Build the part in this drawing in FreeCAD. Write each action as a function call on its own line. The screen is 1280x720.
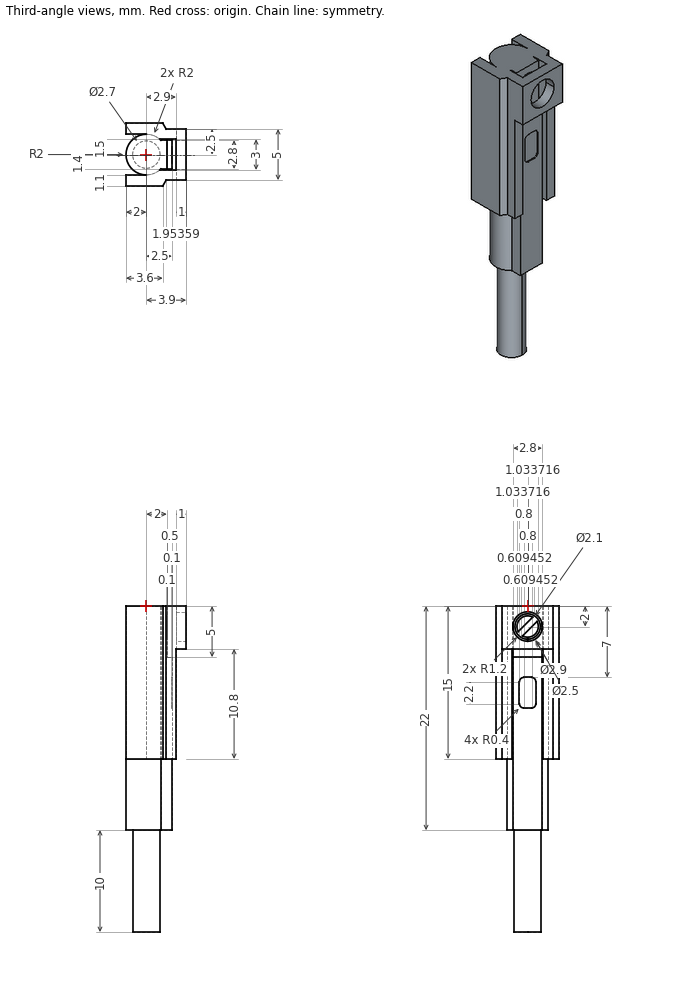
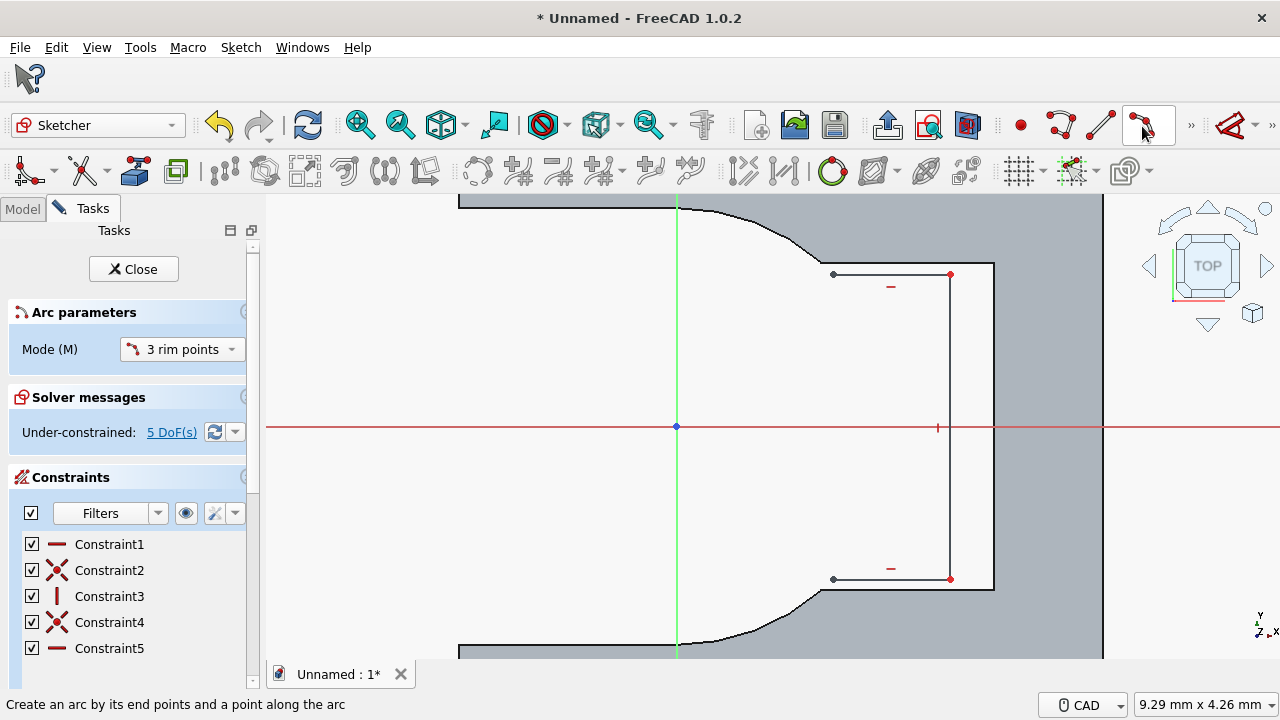
click(833, 275)
click(833, 580)
click(483, 327)
key(Escape)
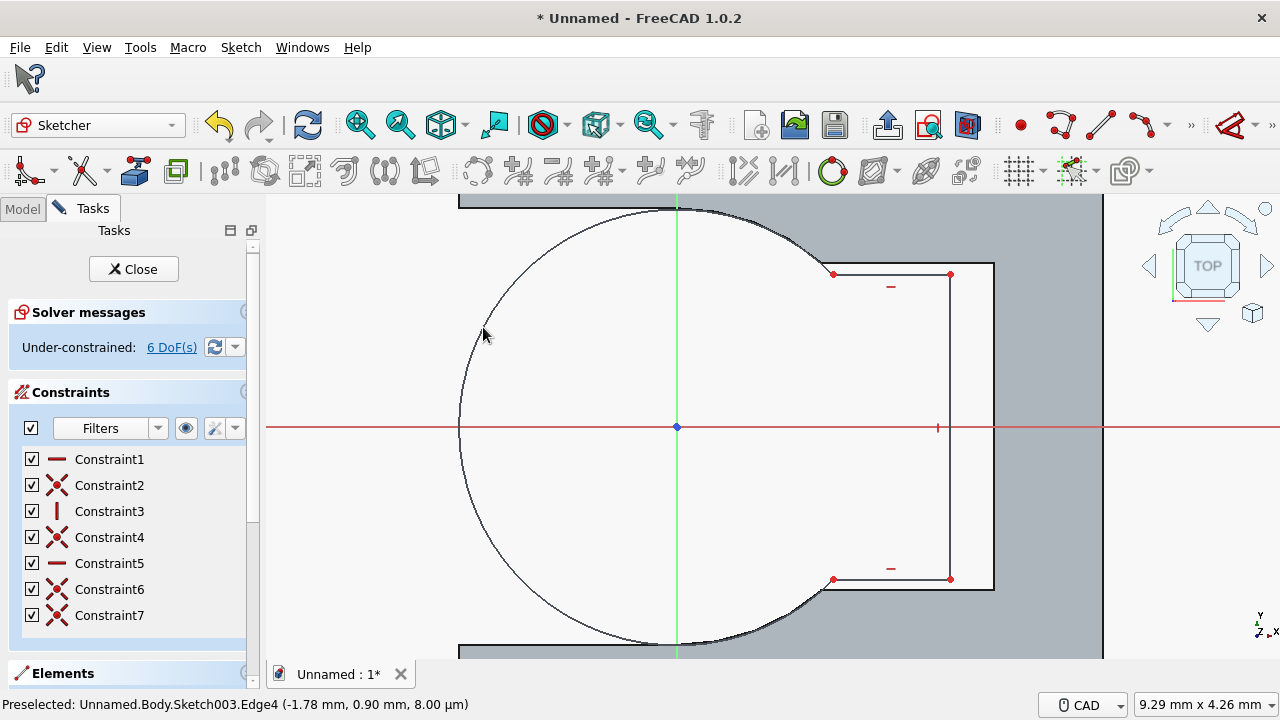
drag(667, 416, 687, 438)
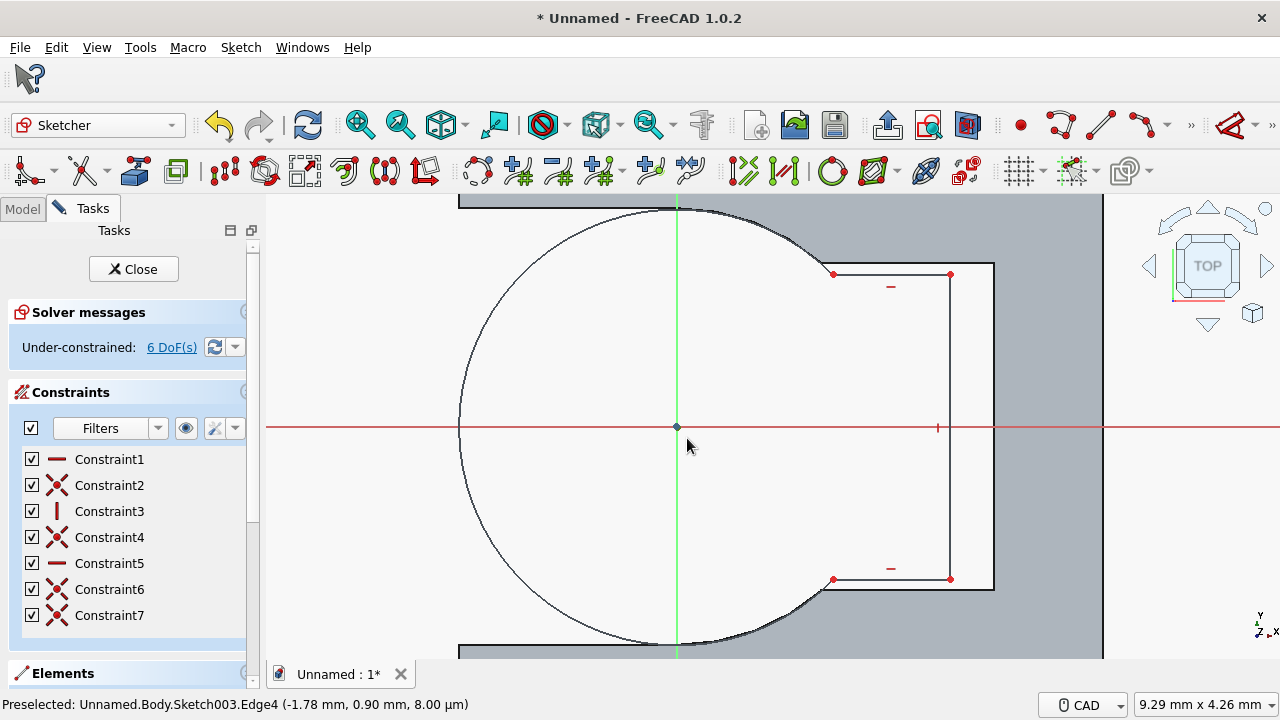
key(c)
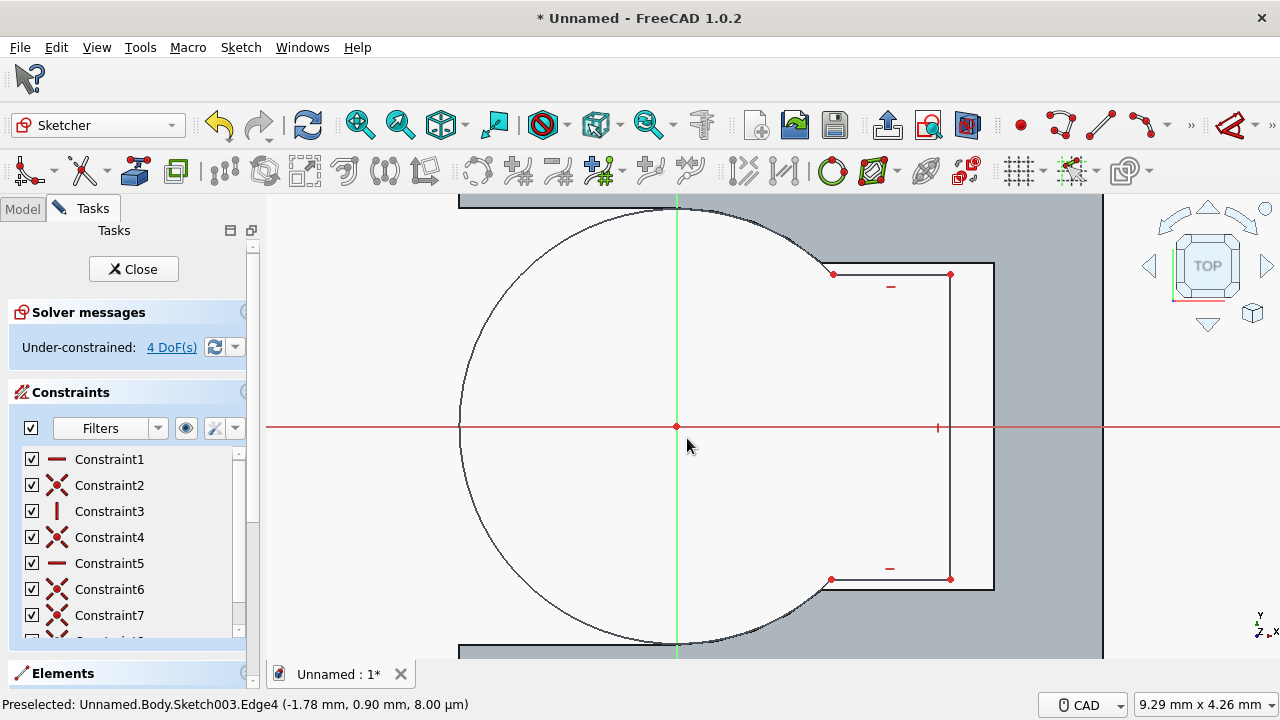
click(1230, 126)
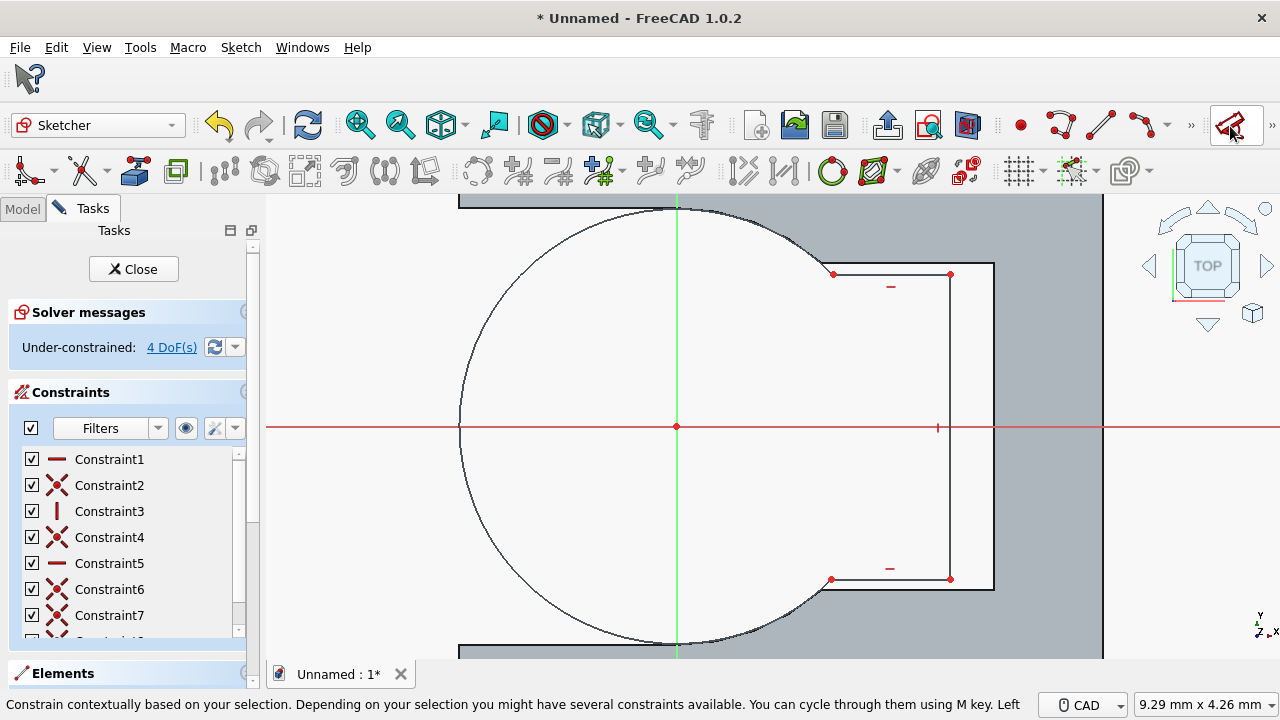
click(551, 249)
click(532, 223)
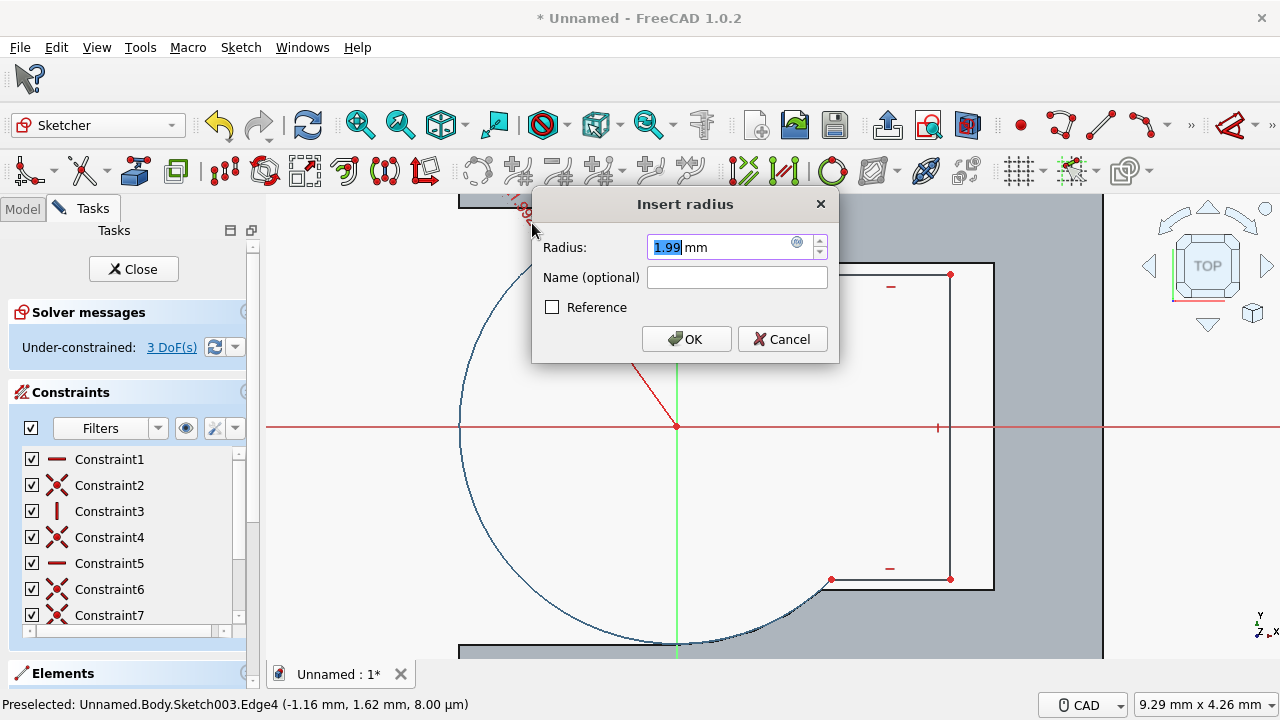
text(2)
key(Return)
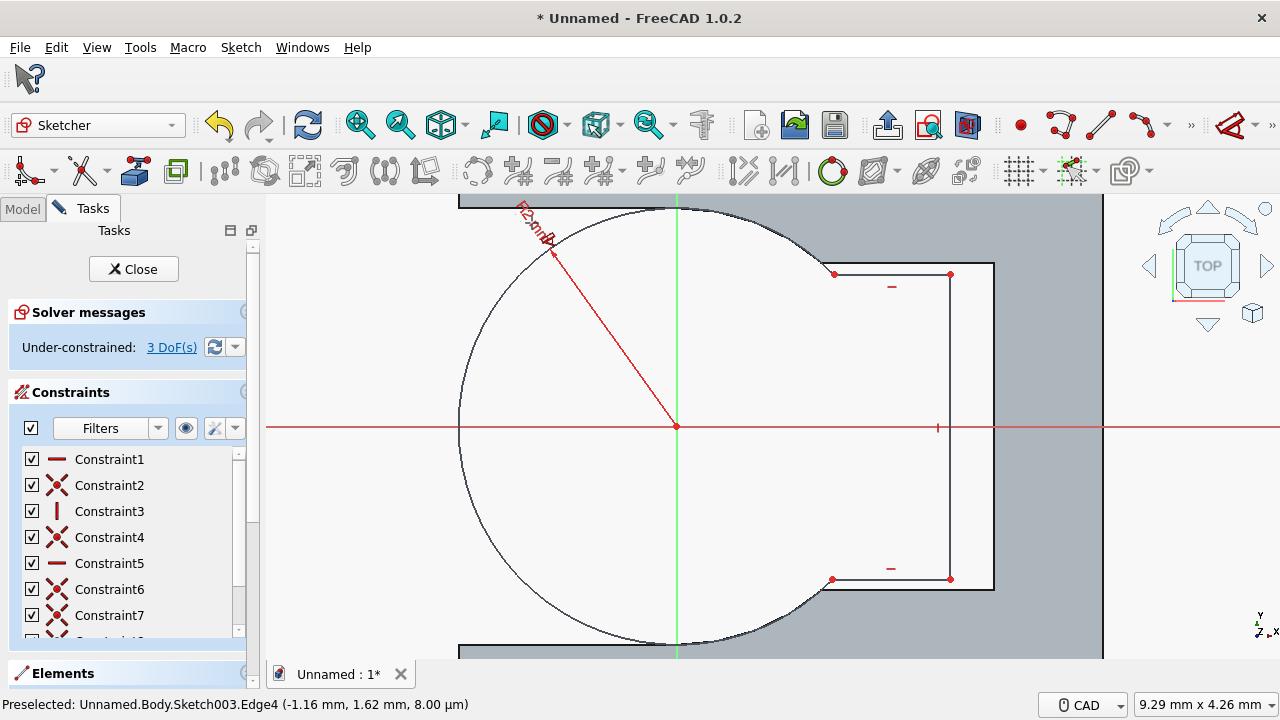
click(950, 489)
click(984, 357)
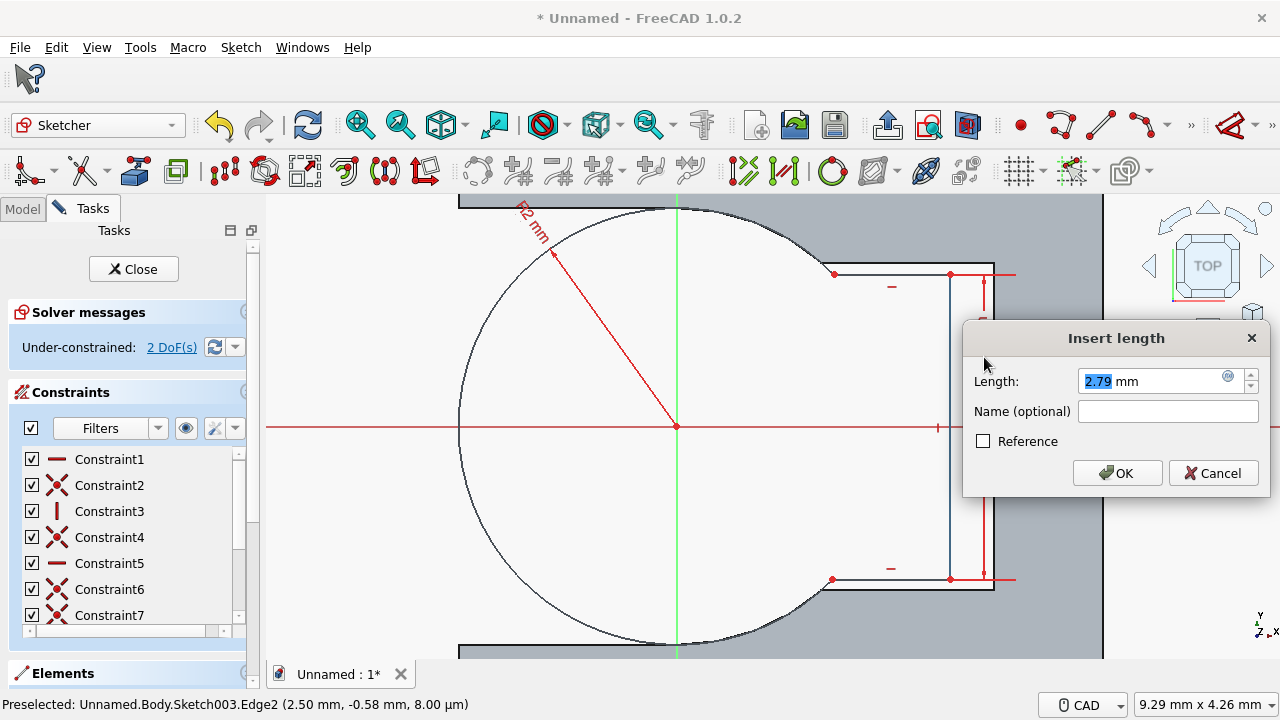
text(2.8)
key(Return)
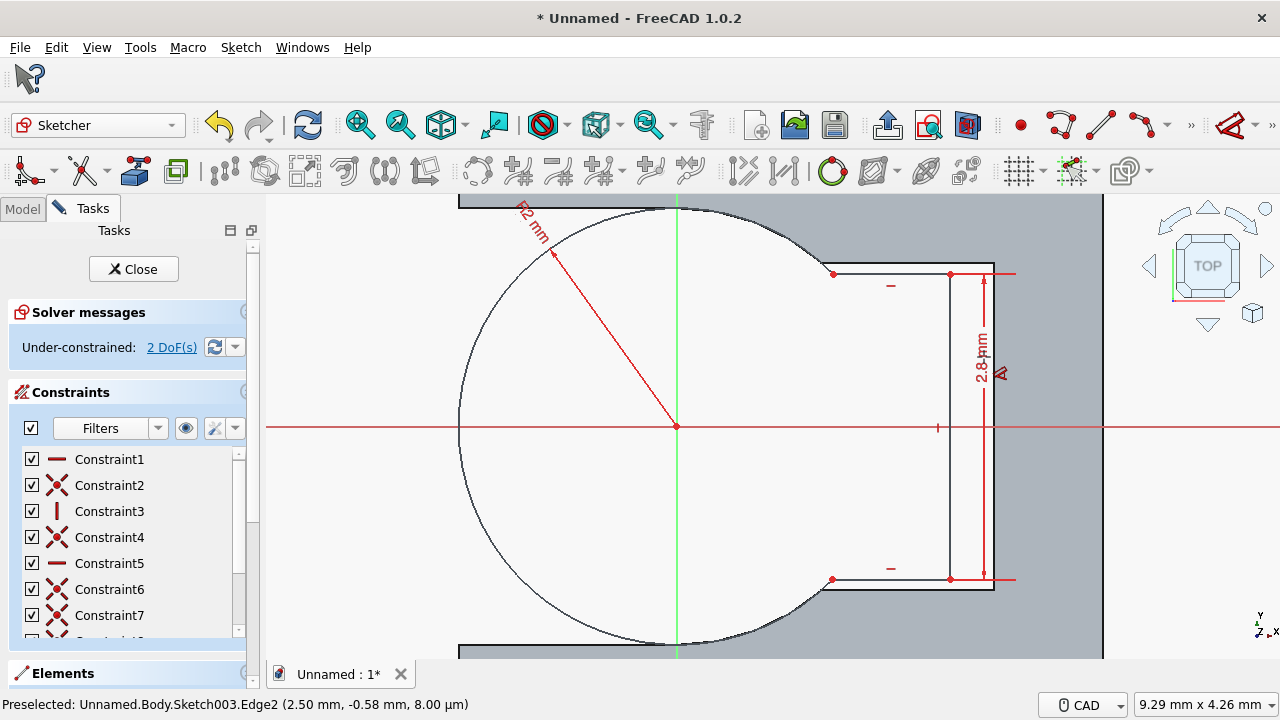
click(832, 580)
click(866, 503)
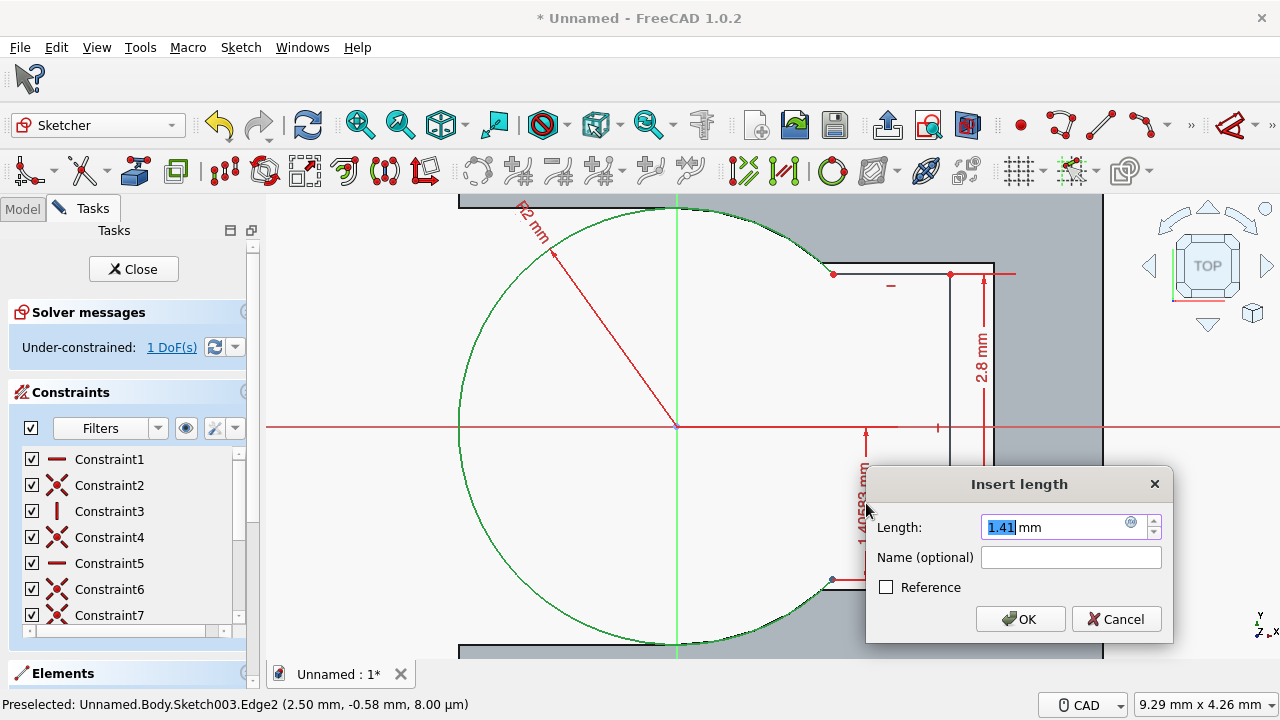
text(1.4)
key(Return)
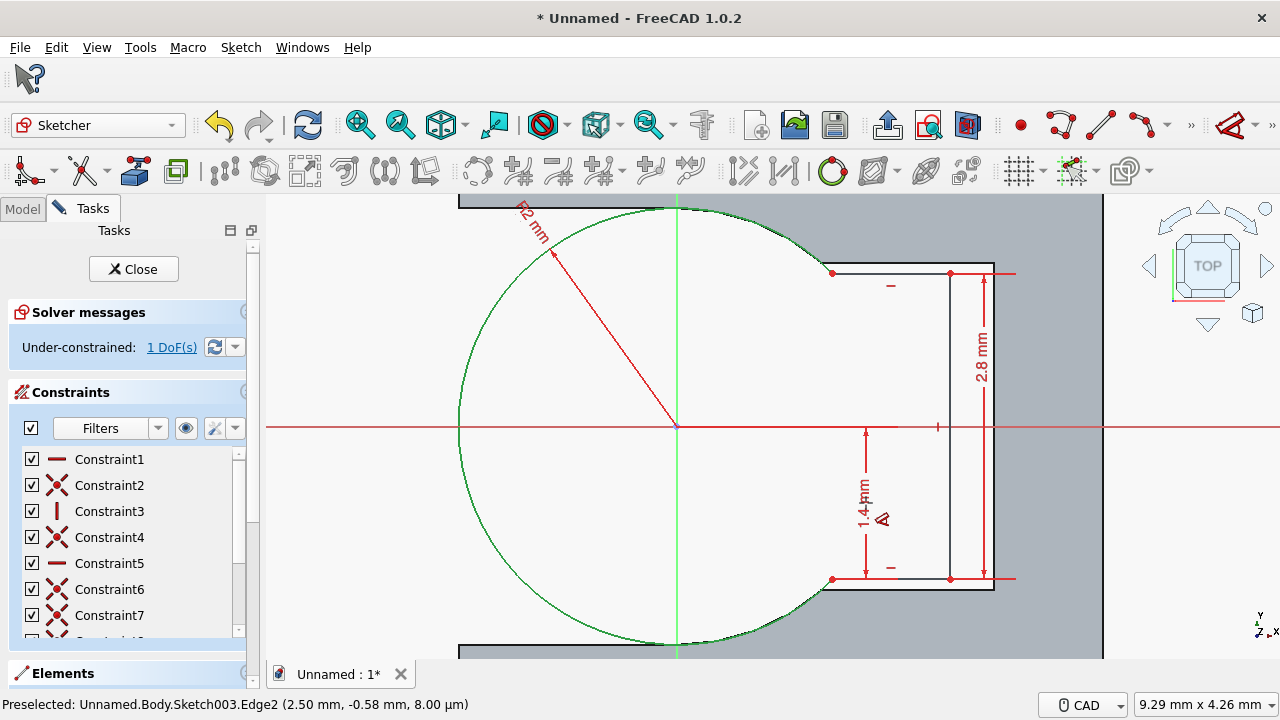
click(950, 579)
click(813, 613)